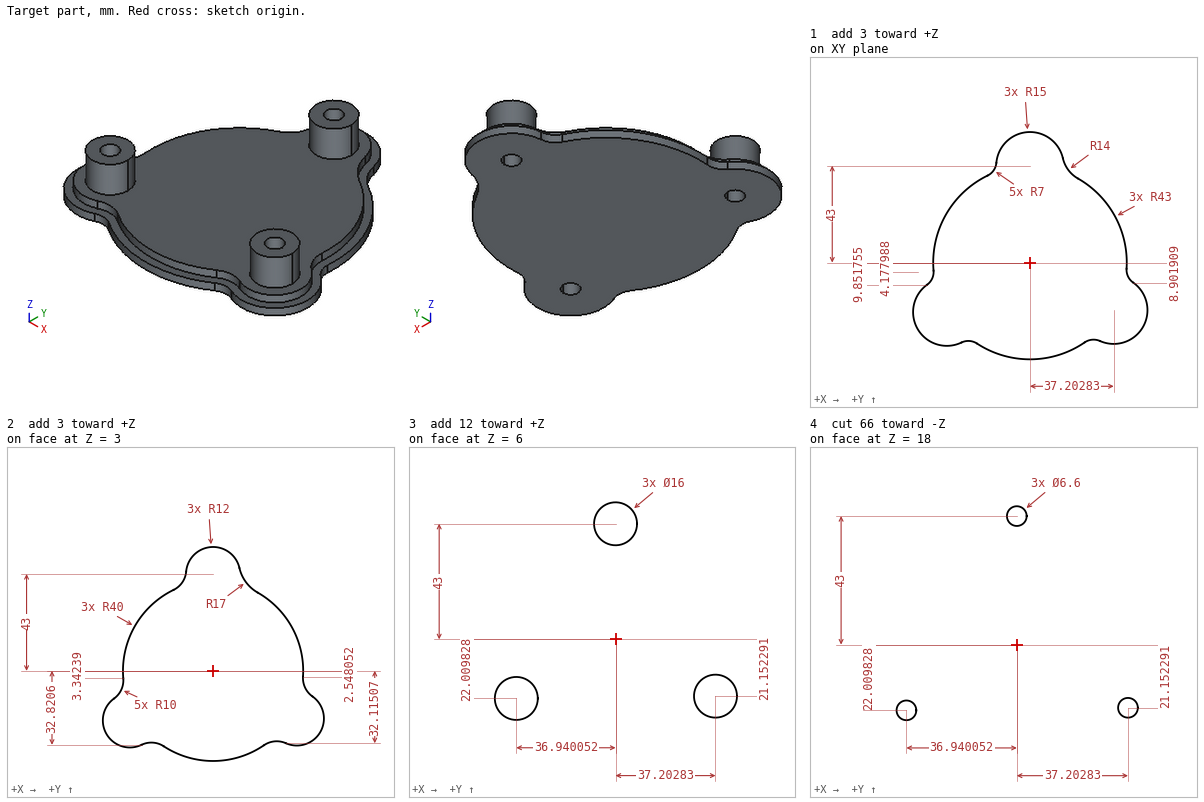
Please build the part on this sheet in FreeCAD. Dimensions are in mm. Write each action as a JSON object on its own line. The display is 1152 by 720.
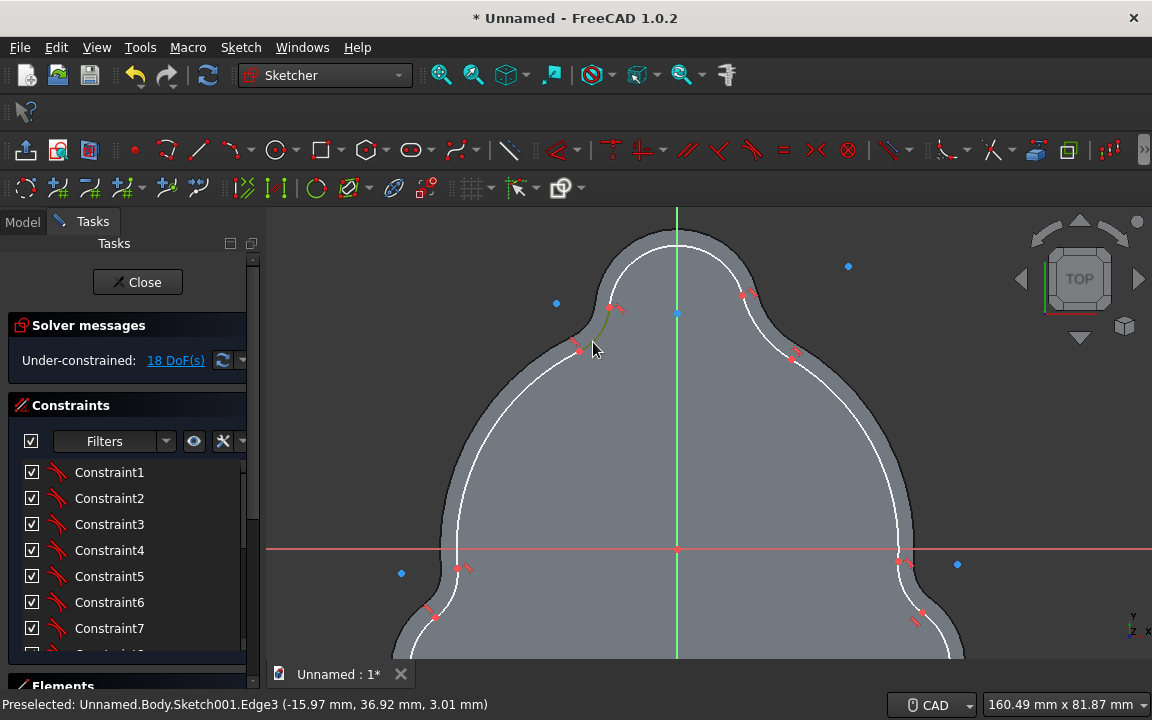
{"action": "left_click", "coordinate": [447, 606]}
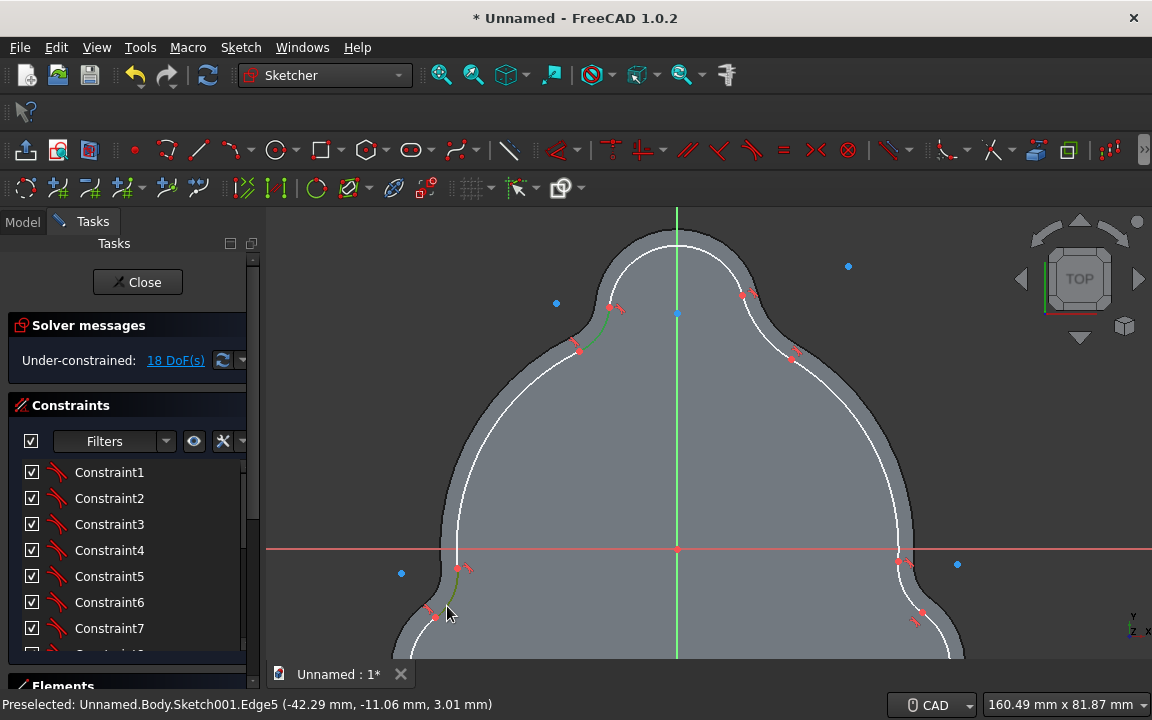
{"action": "scroll", "coordinate": [594, 342], "scroll_direction": "down", "scroll_amount": 3}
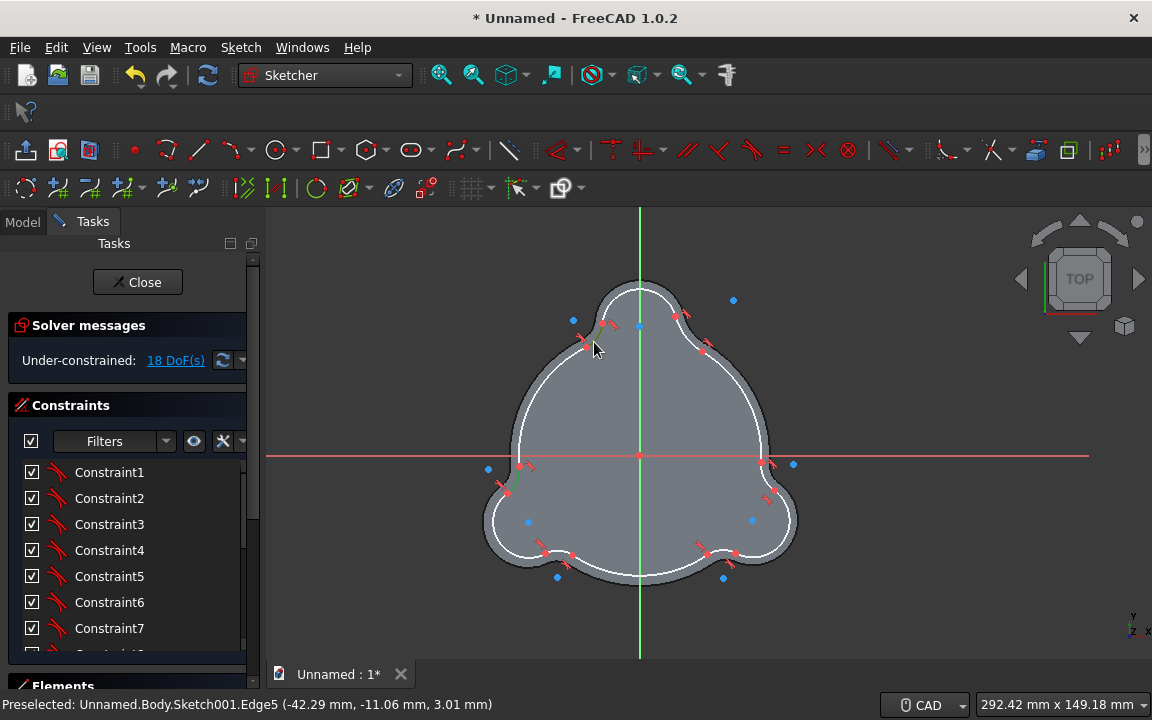
{"action": "scroll", "coordinate": [565, 552], "scroll_direction": "up", "scroll_amount": 3}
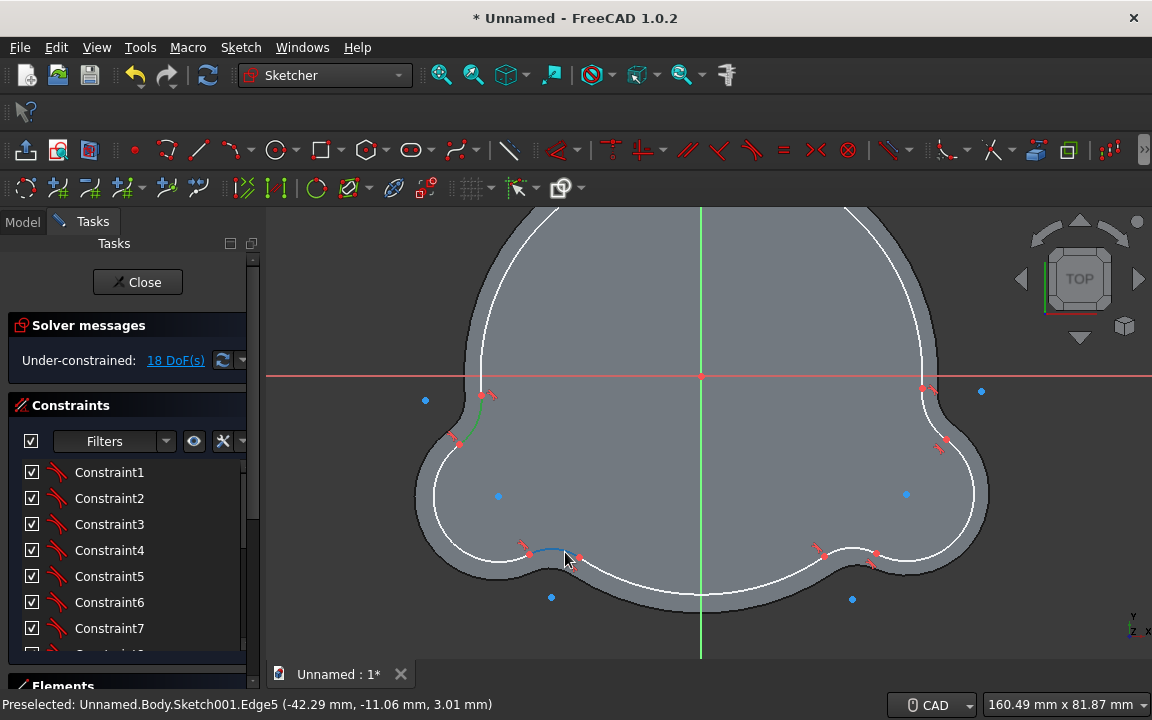
{"action": "left_click", "coordinate": [565, 551]}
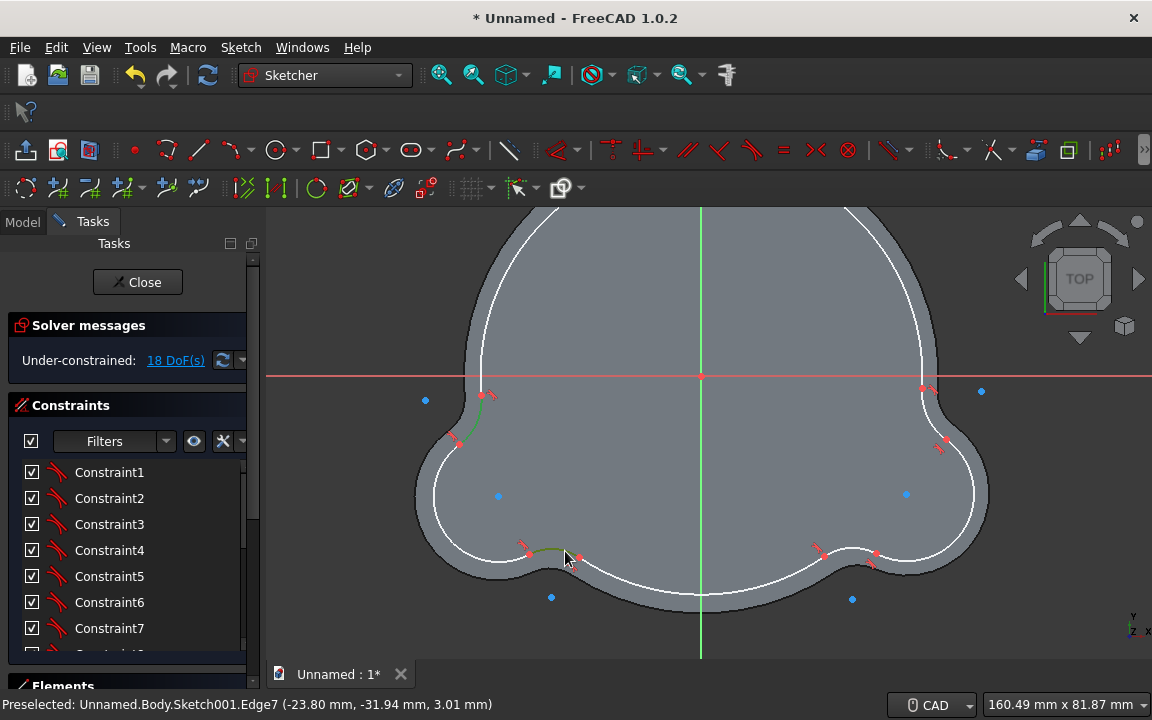
{"action": "left_click", "coordinate": [861, 549]}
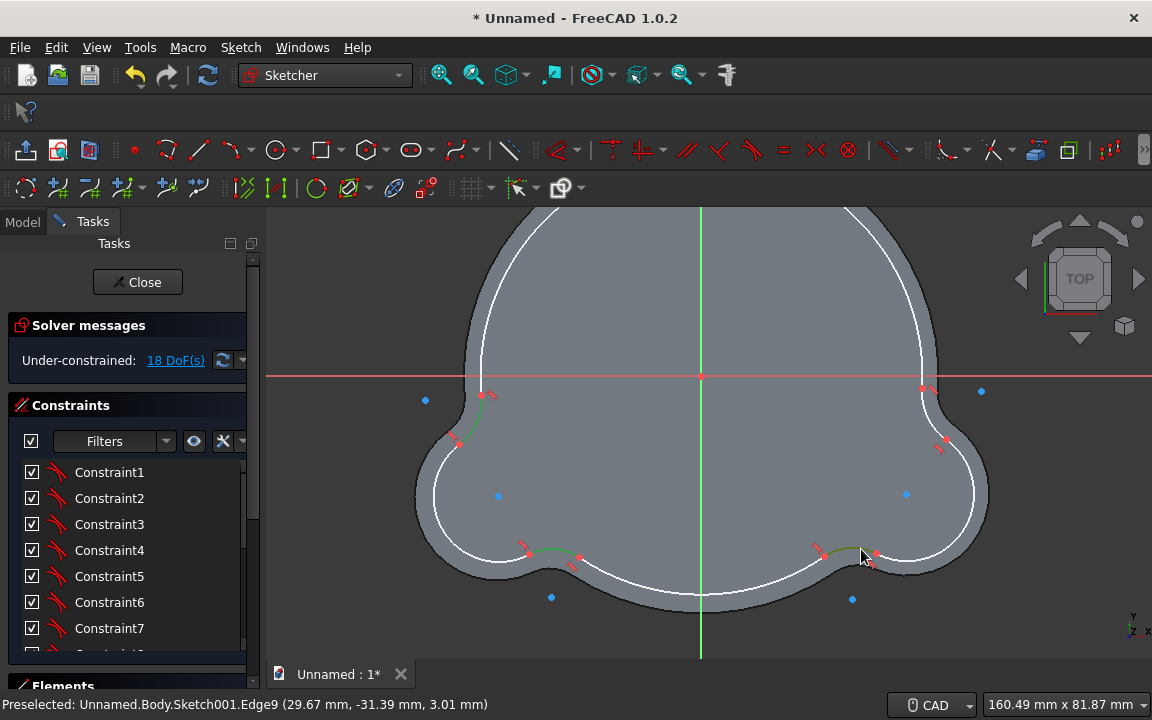
{"action": "left_click", "coordinate": [924, 406]}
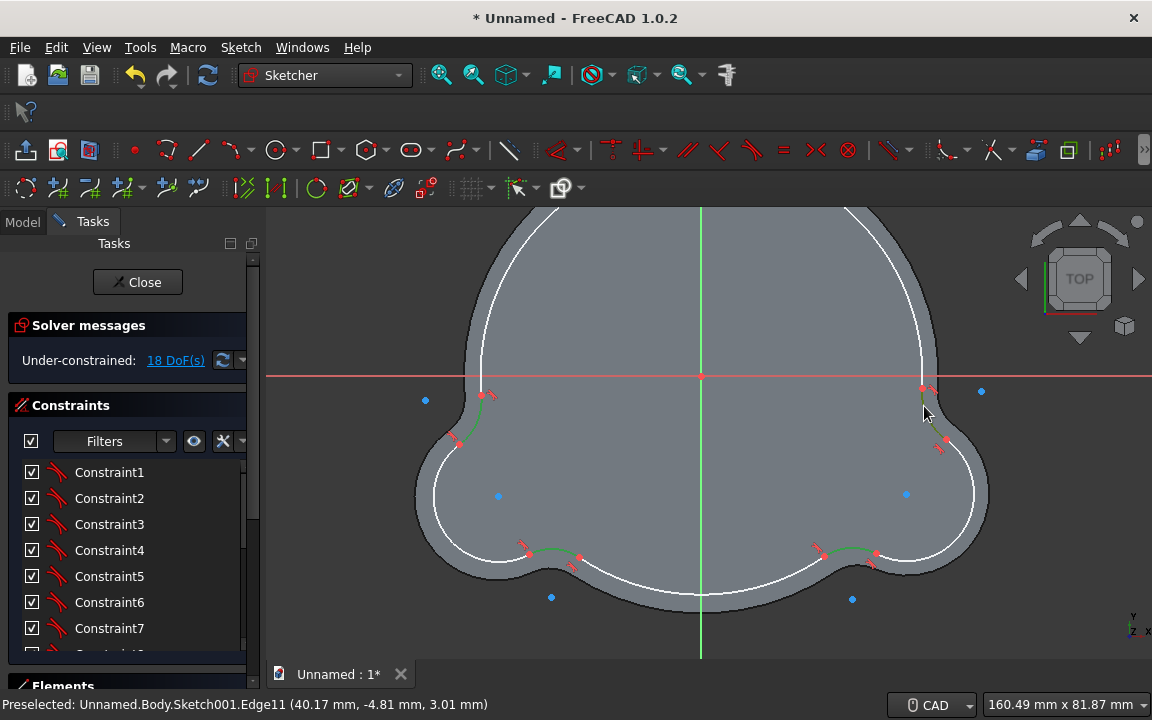
{"action": "left_click", "coordinate": [784, 150]}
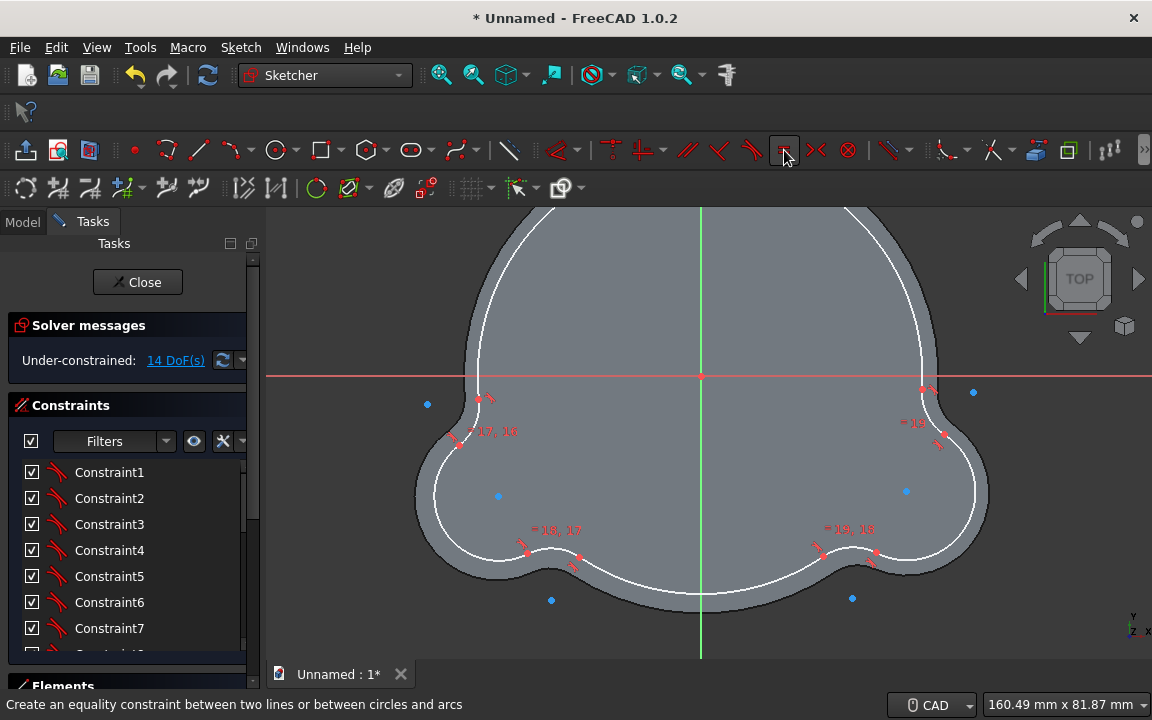
{"action": "scroll", "coordinate": [565, 552], "scroll_direction": "down", "scroll_amount": 3}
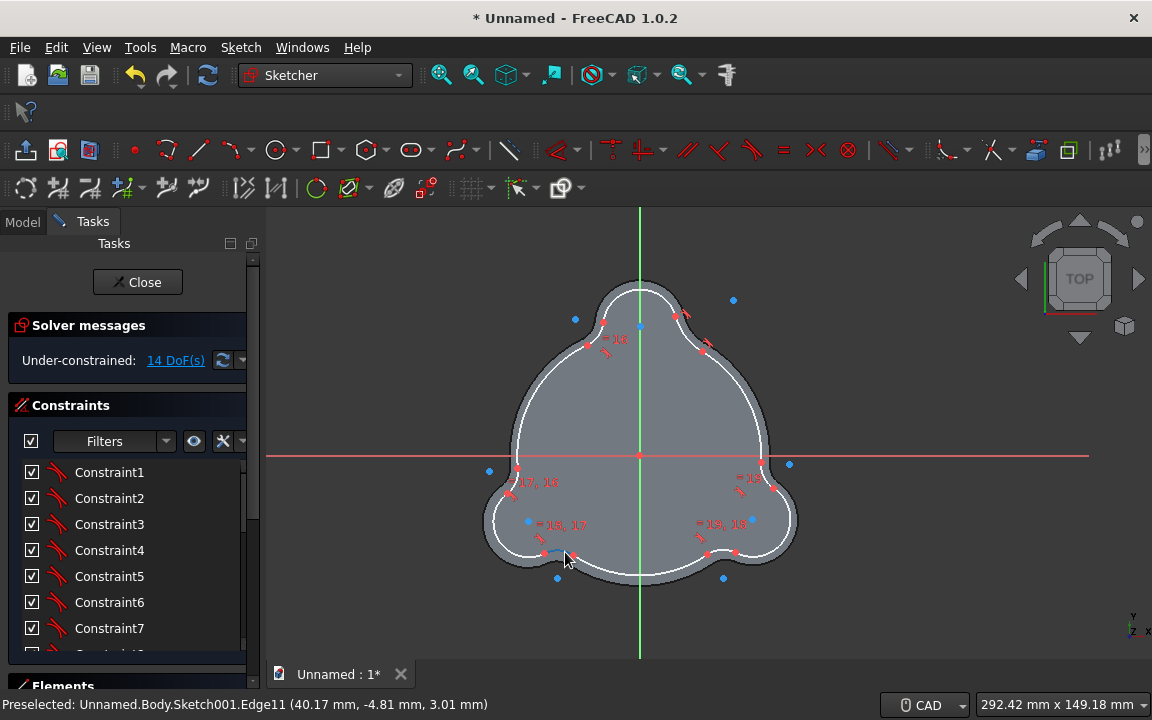
{"action": "left_click", "coordinate": [657, 294]}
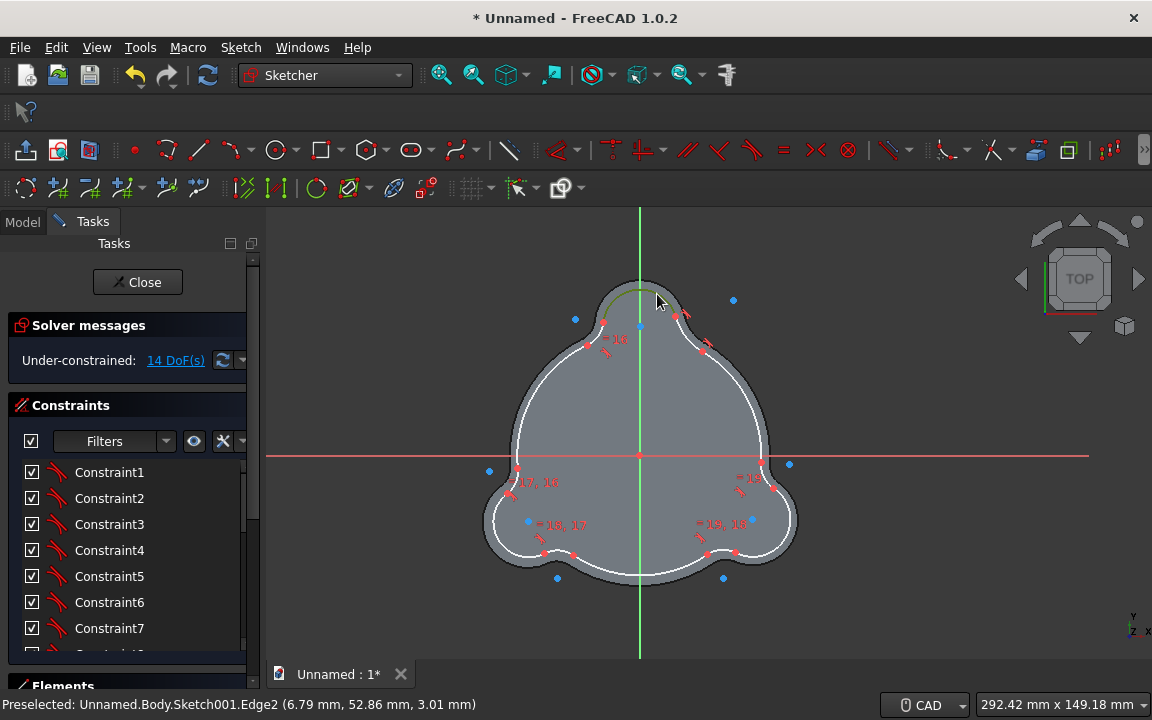
{"action": "left_click", "coordinate": [493, 521]}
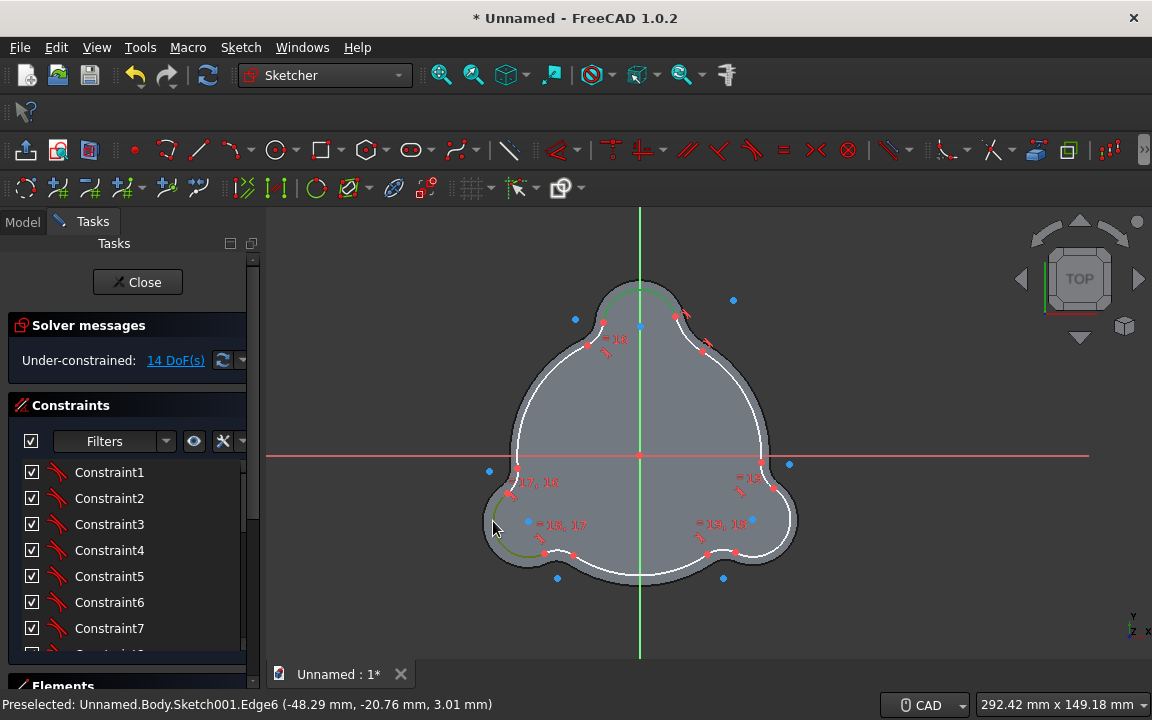
{"action": "left_click", "coordinate": [769, 553]}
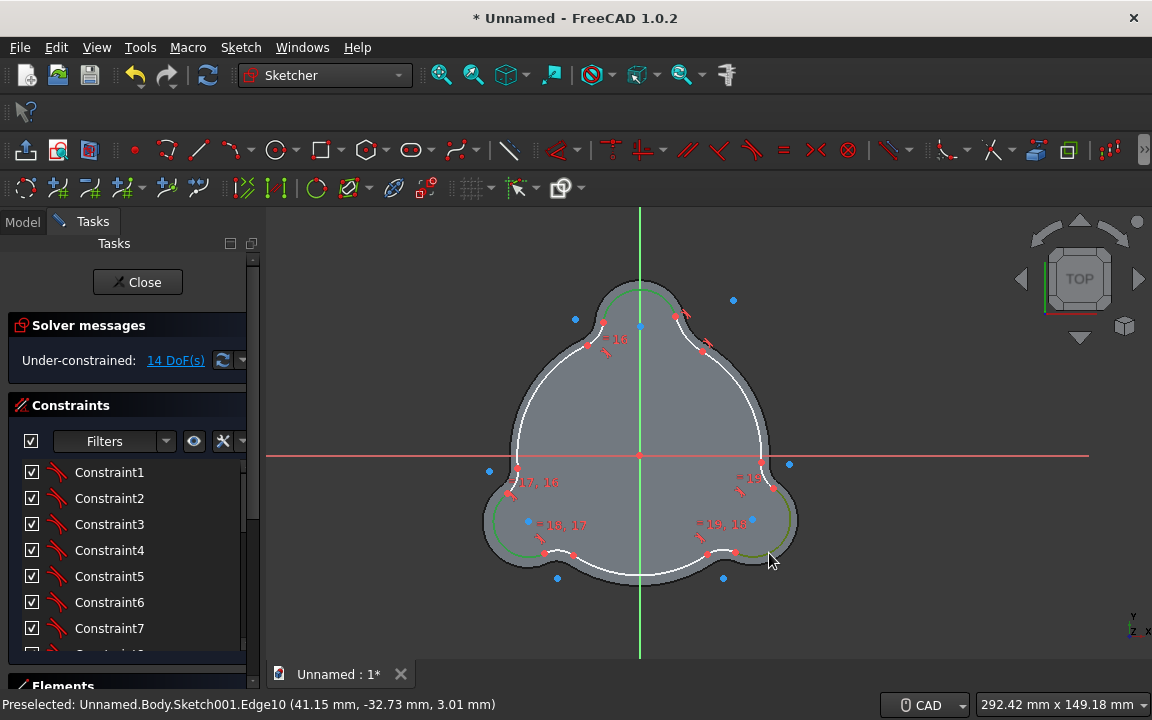
{"action": "left_click", "coordinate": [784, 150]}